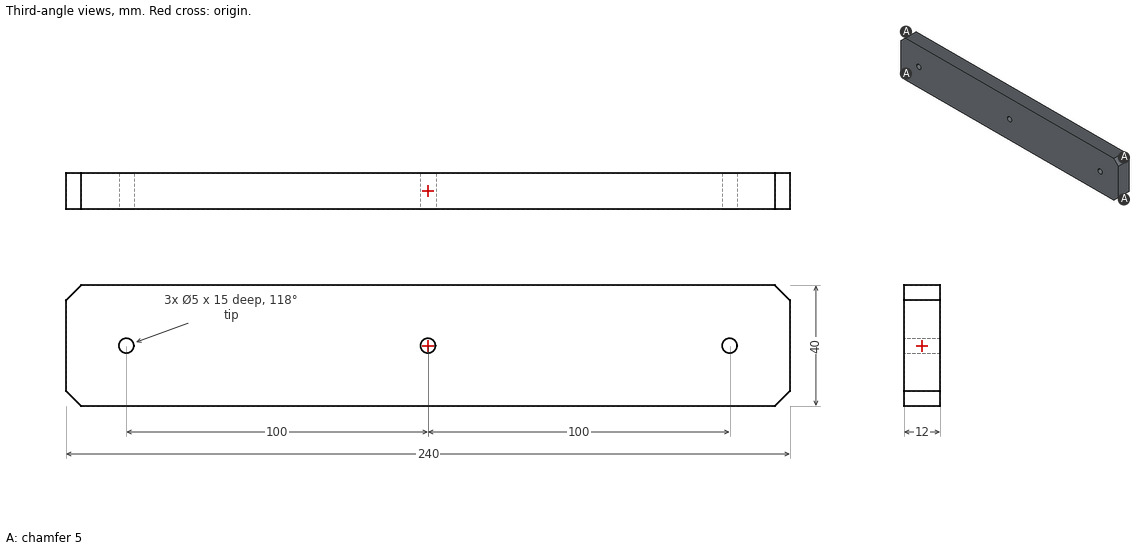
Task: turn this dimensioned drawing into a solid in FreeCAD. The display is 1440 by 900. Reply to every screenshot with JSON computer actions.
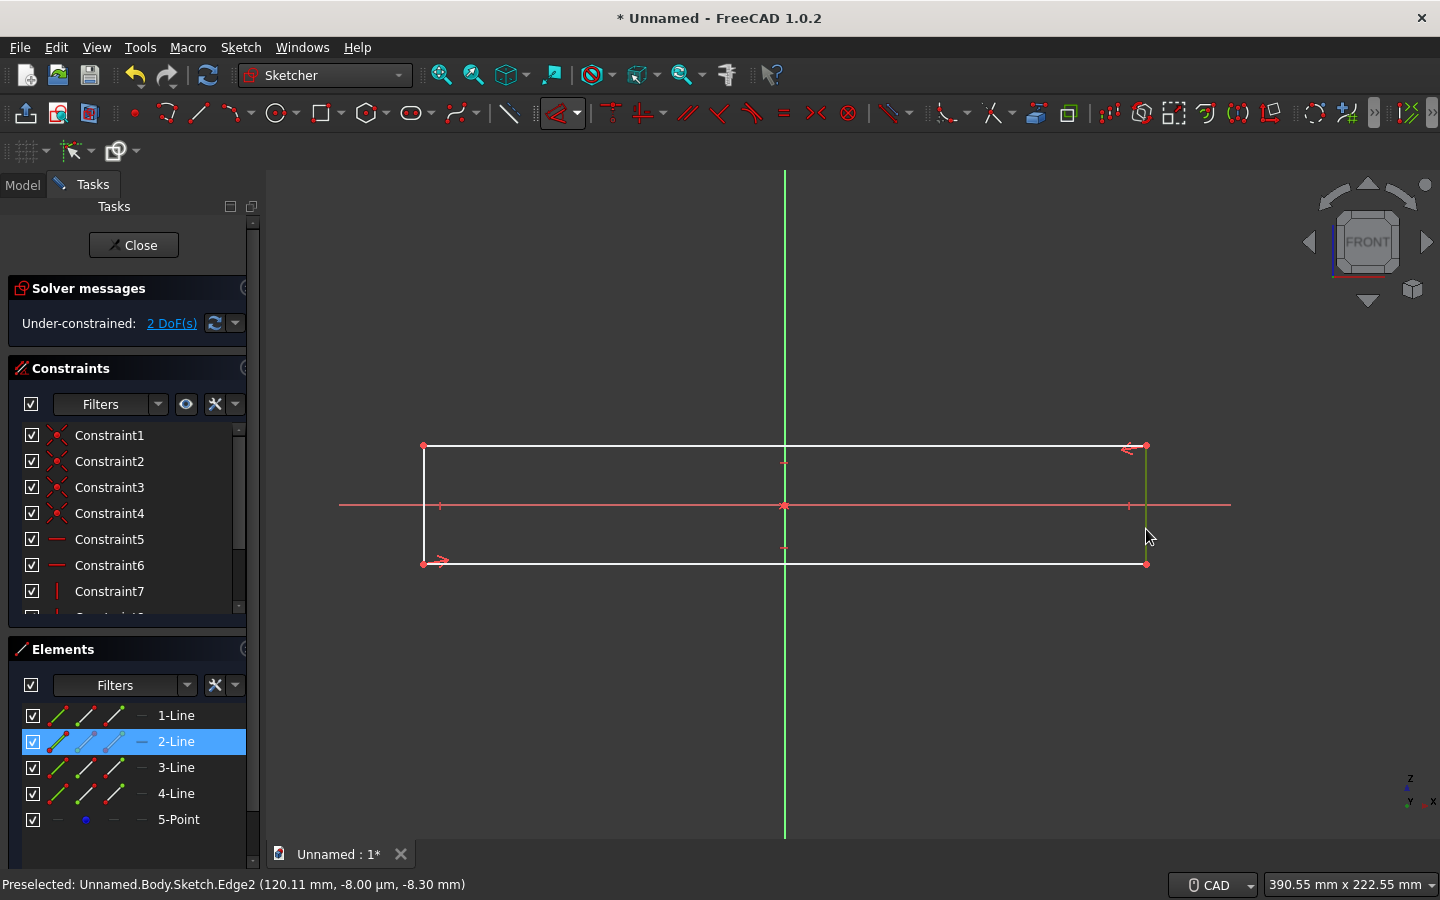
{"action": "left_click", "coordinate": [580, 114]}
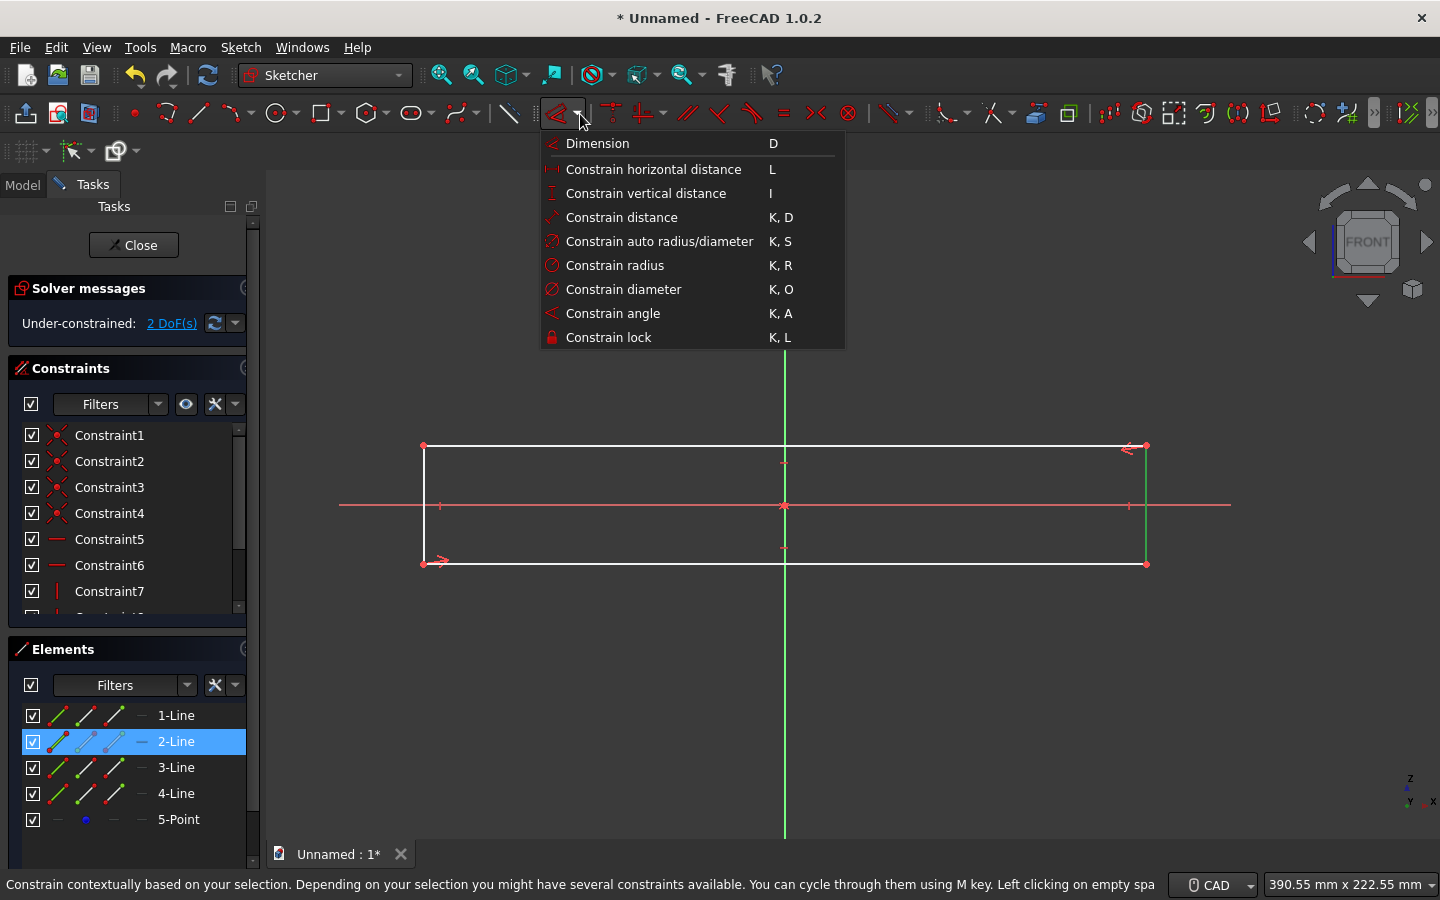
{"action": "left_click", "coordinate": [693, 193]}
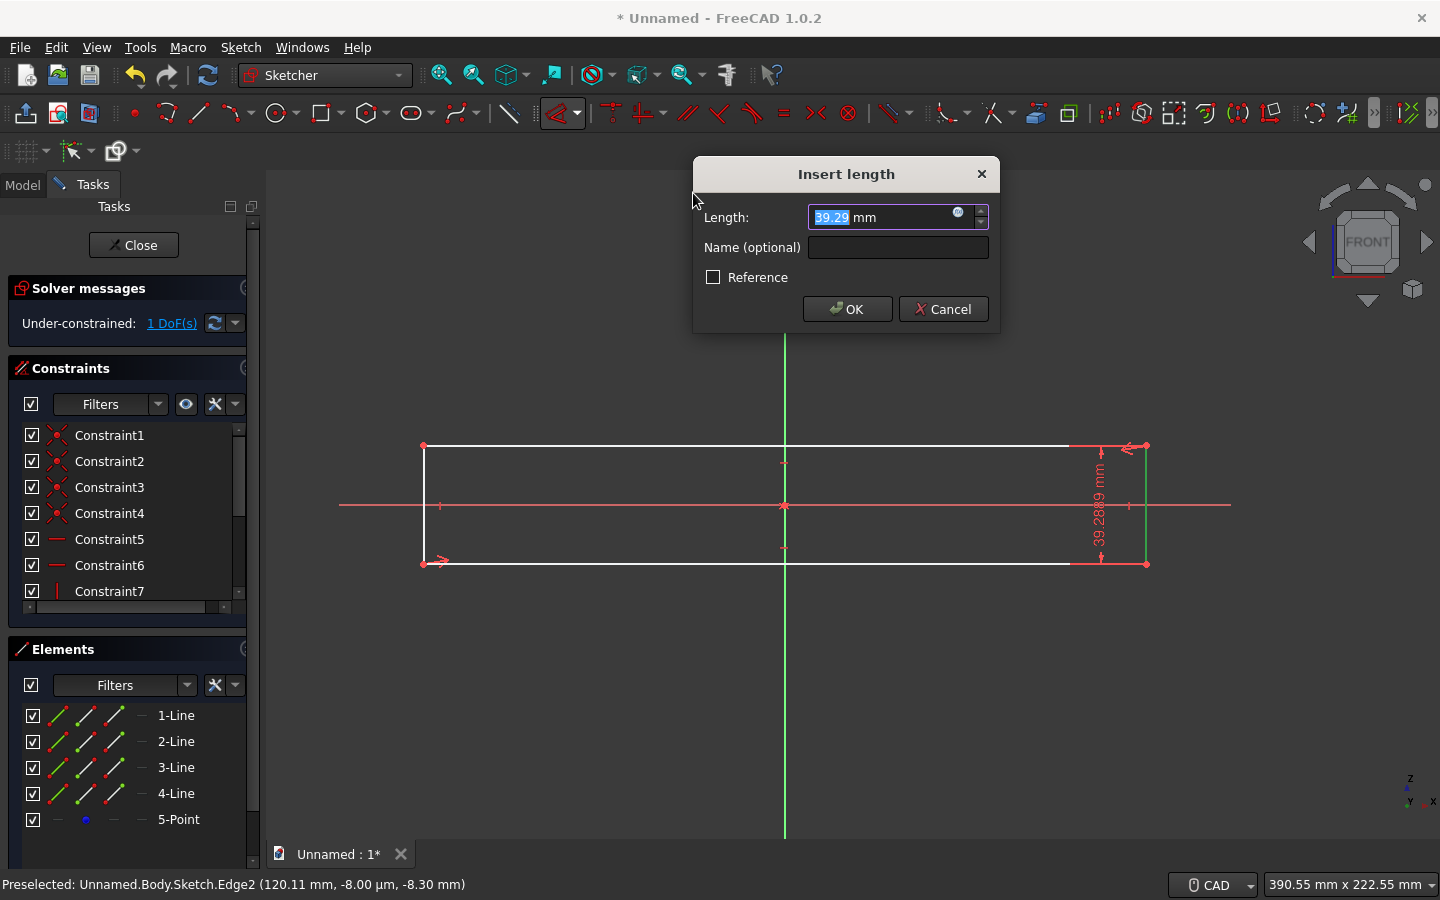
{"action": "type", "text": "40"}
{"action": "key", "text": "Return"}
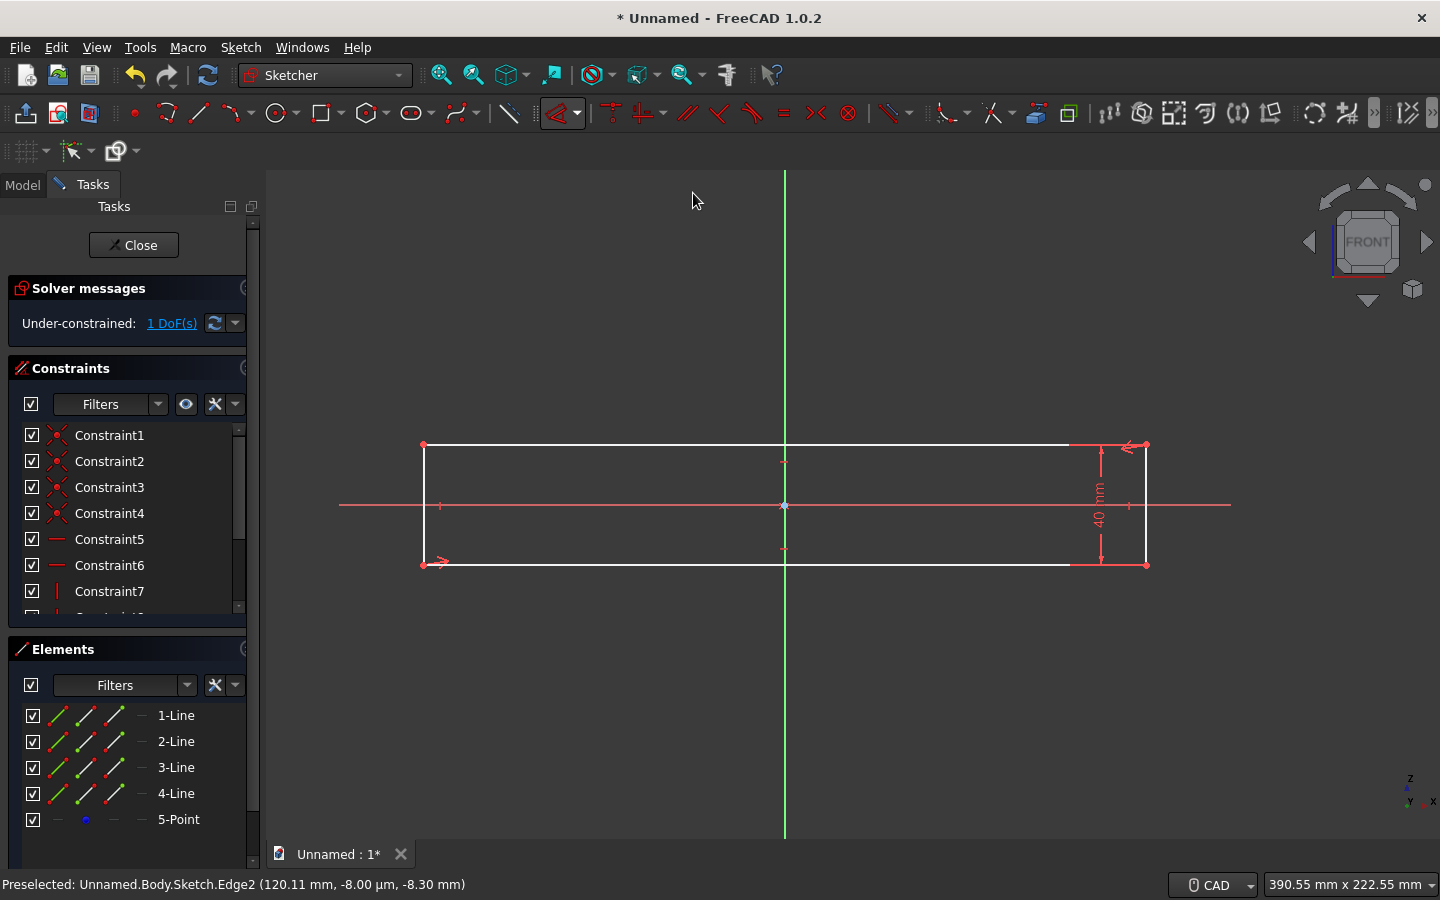
{"action": "left_click", "coordinate": [641, 565]}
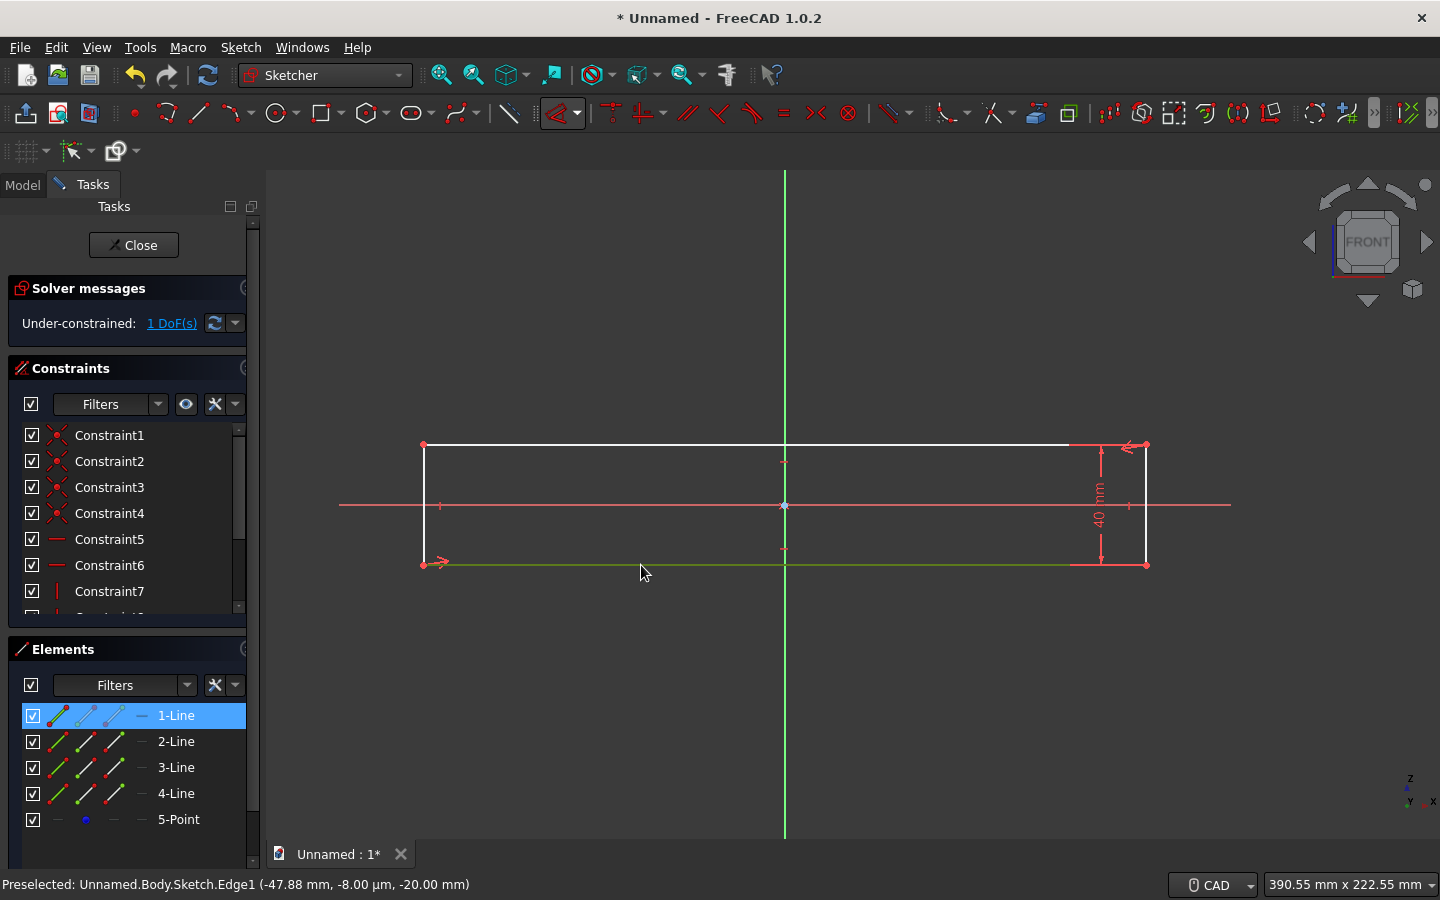
{"action": "left_click", "coordinate": [580, 114]}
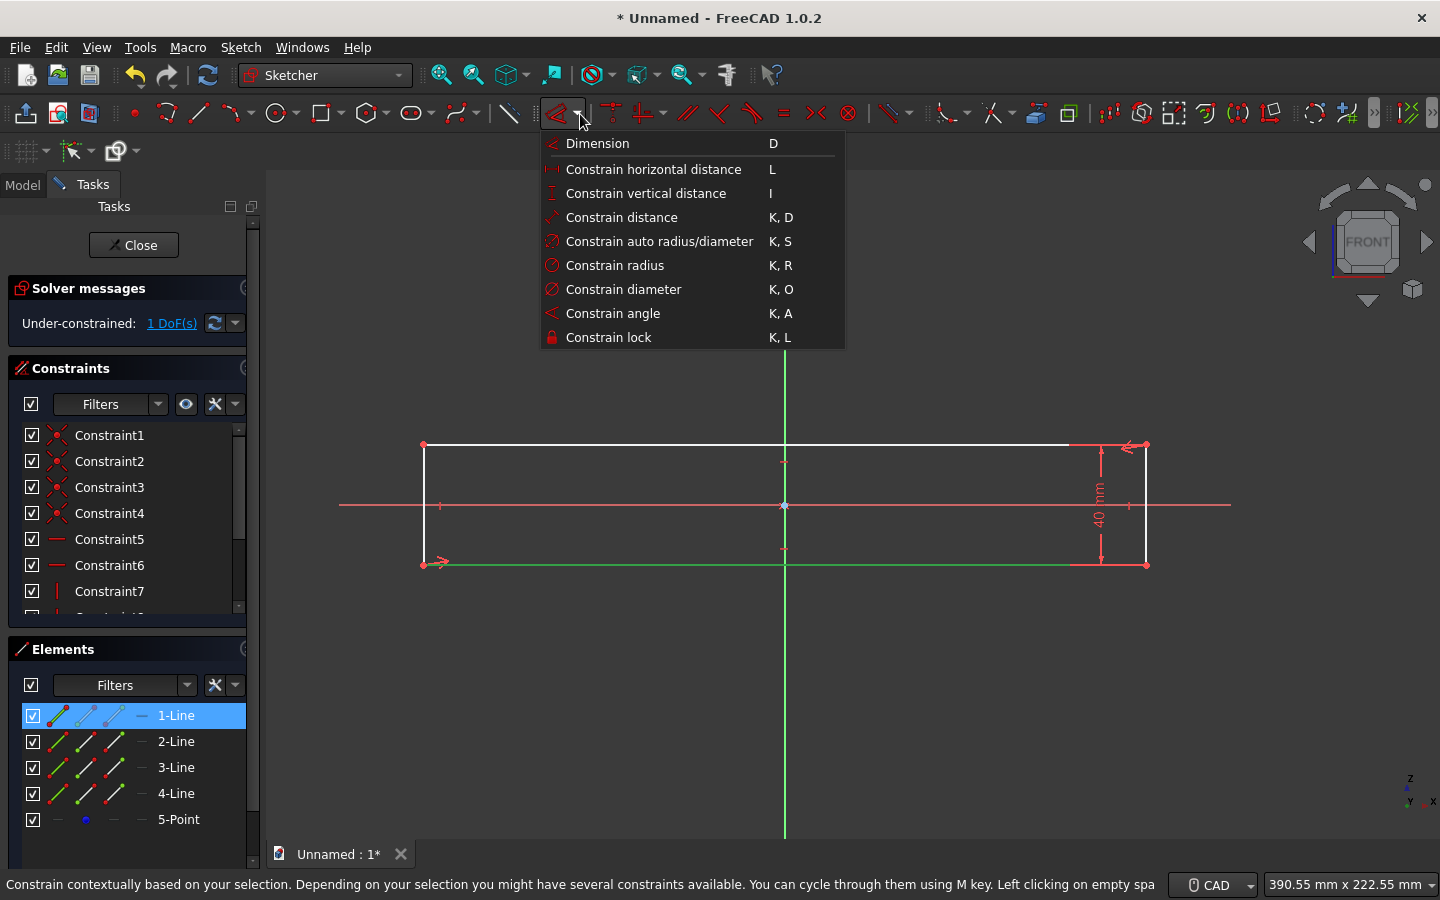
{"action": "left_click", "coordinate": [693, 169]}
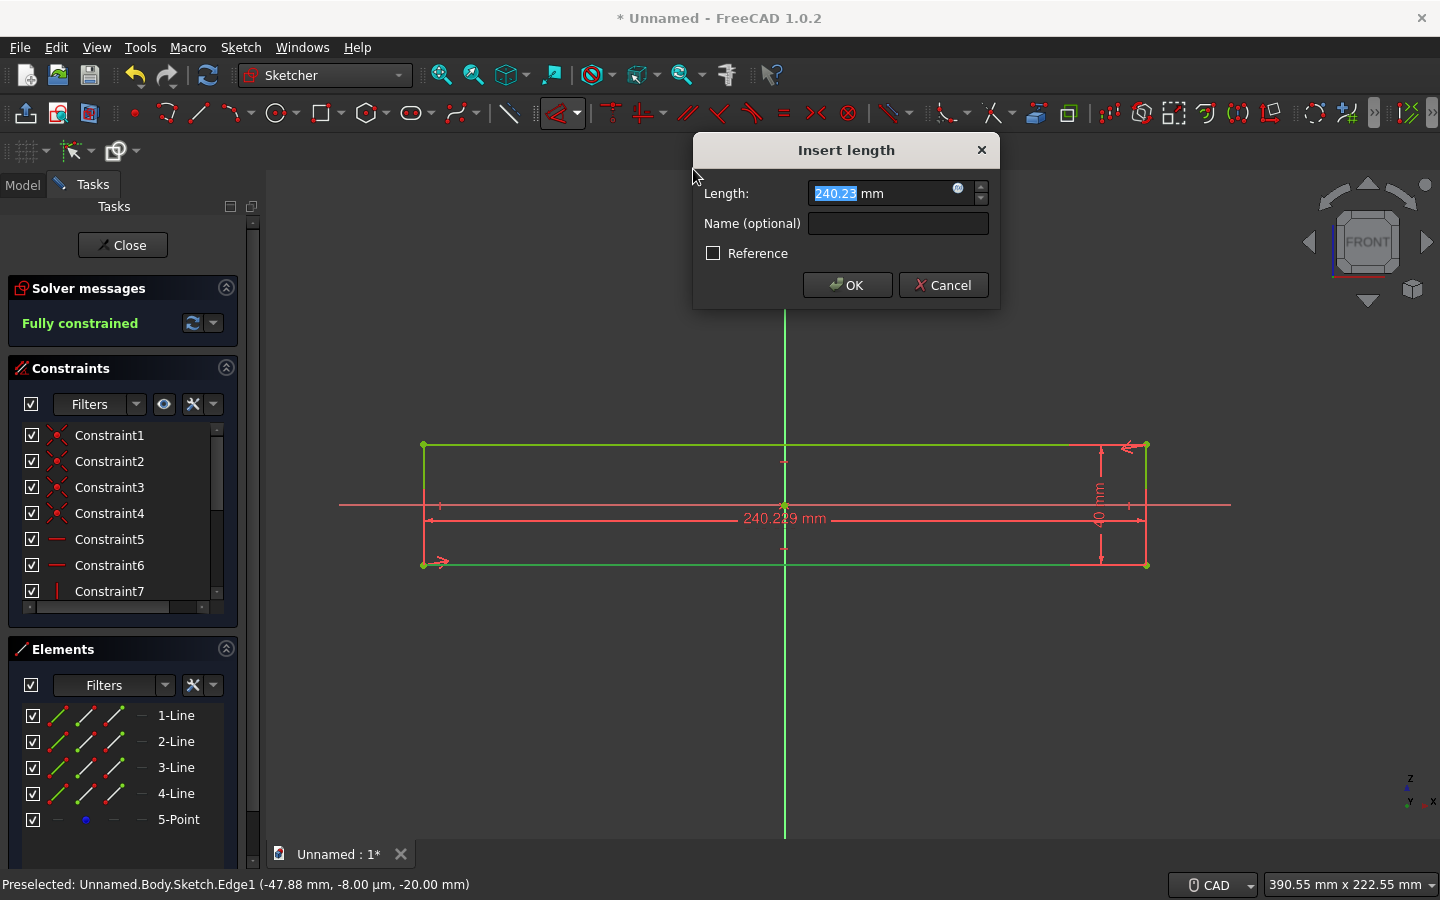
{"action": "type", "text": "240"}
{"action": "key", "text": "Return"}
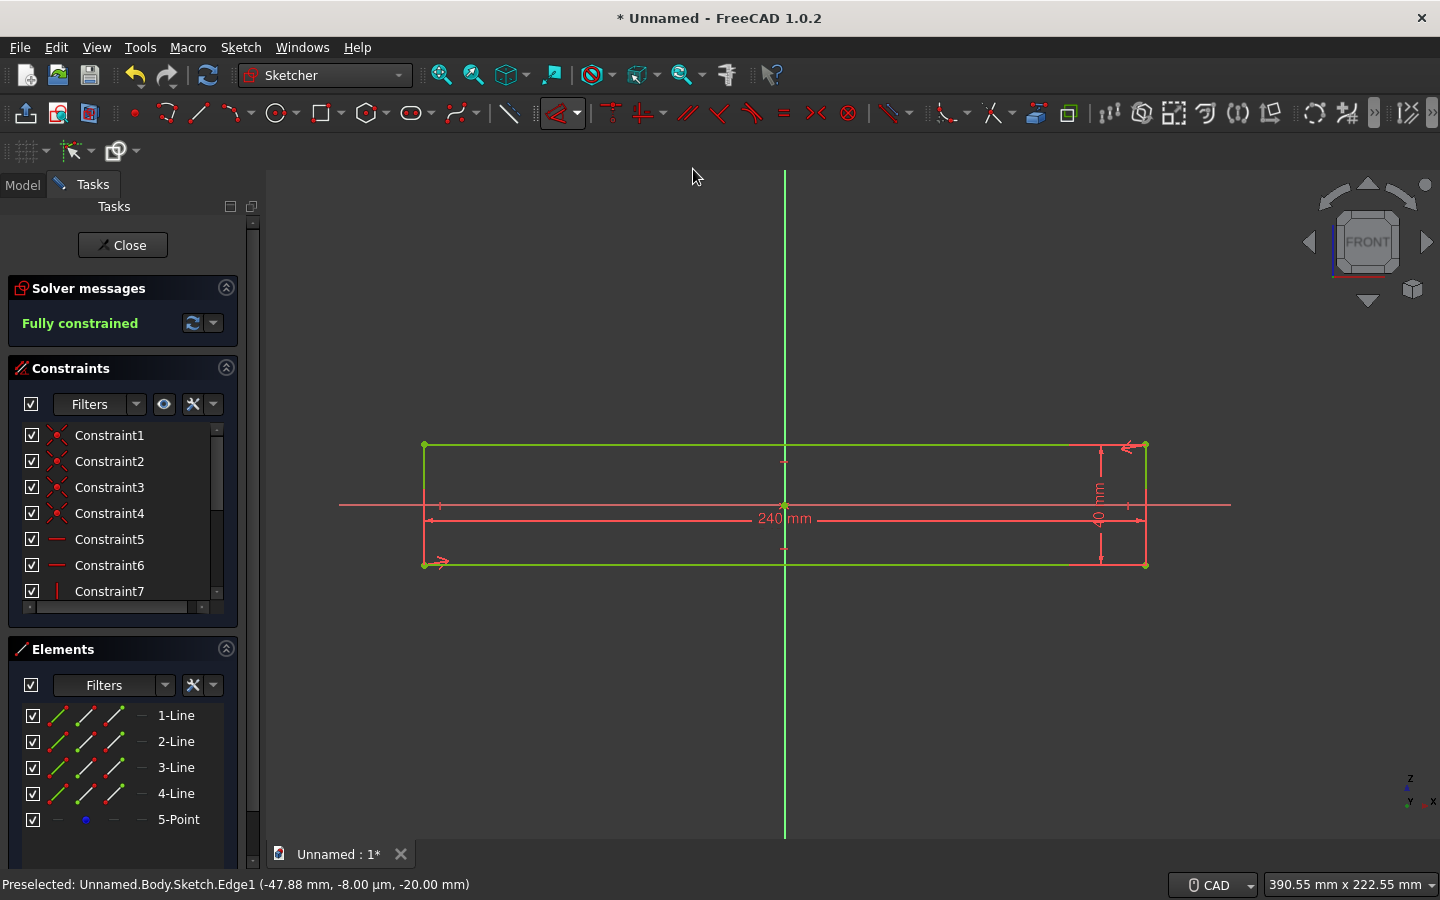
{"action": "left_click", "coordinate": [123, 245]}